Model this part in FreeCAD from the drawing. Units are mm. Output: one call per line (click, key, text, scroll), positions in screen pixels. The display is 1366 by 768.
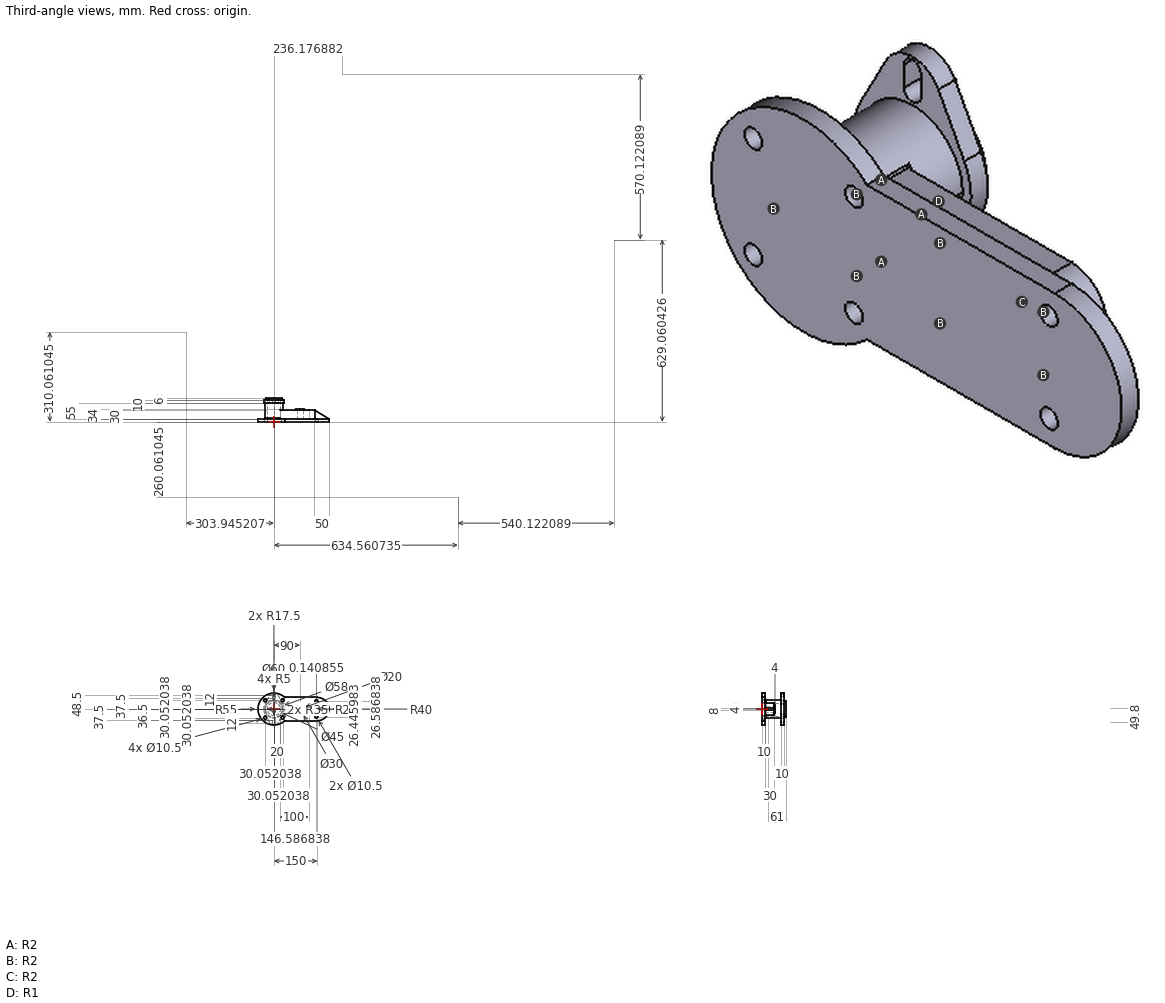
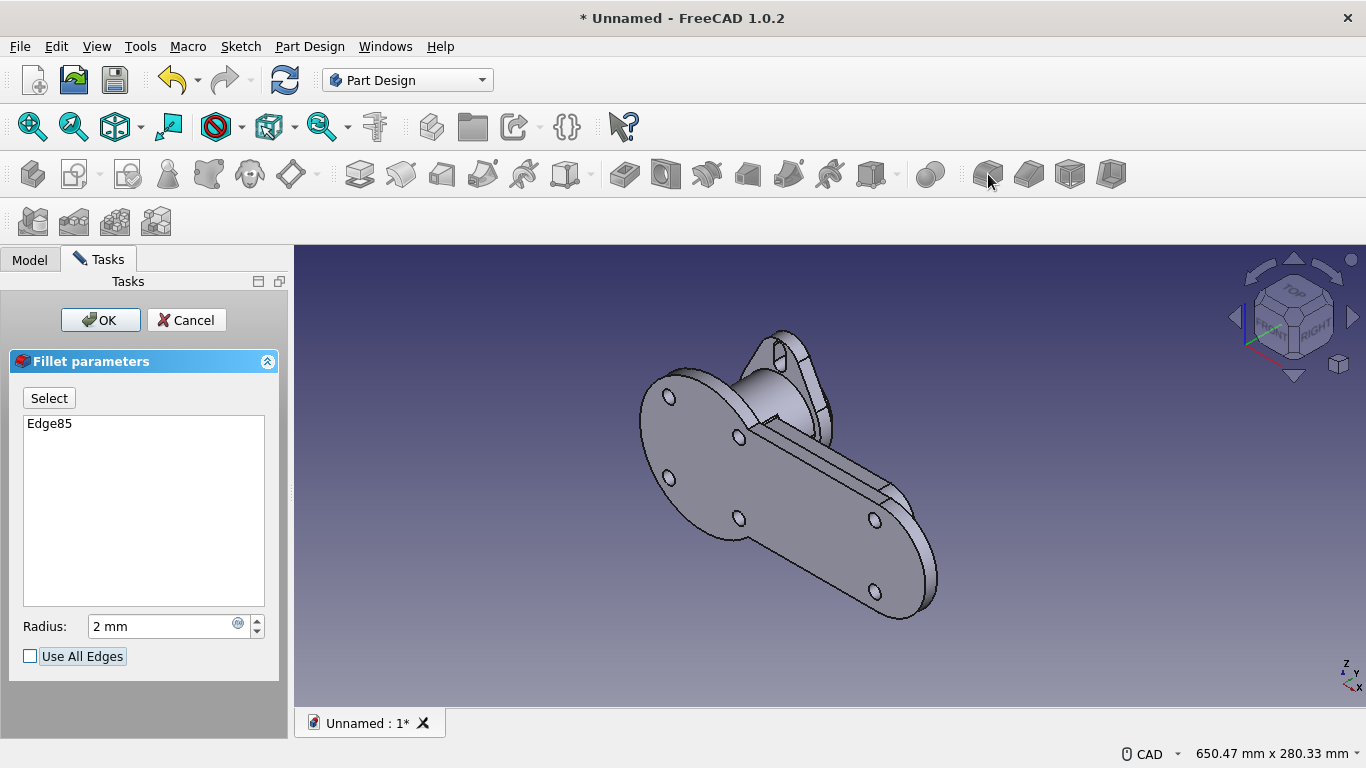
click(101, 320)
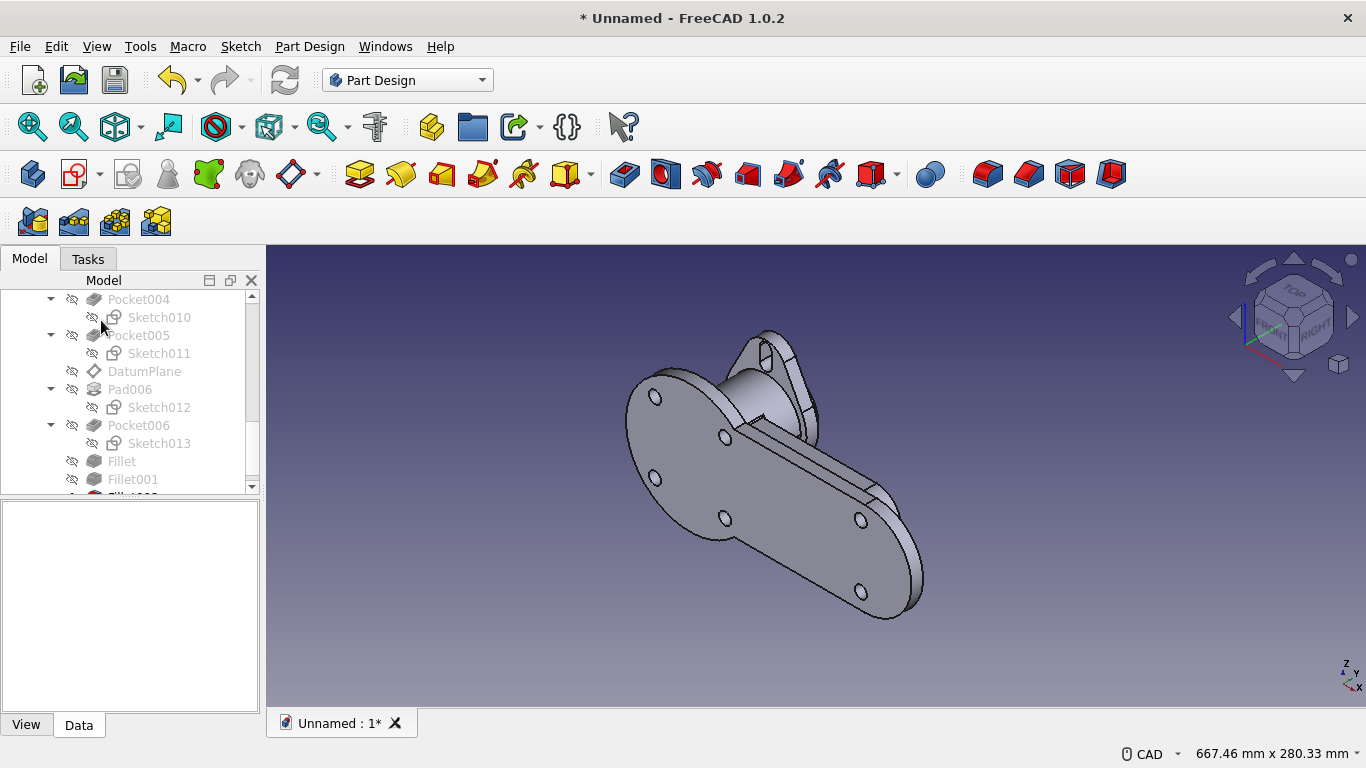
key(2)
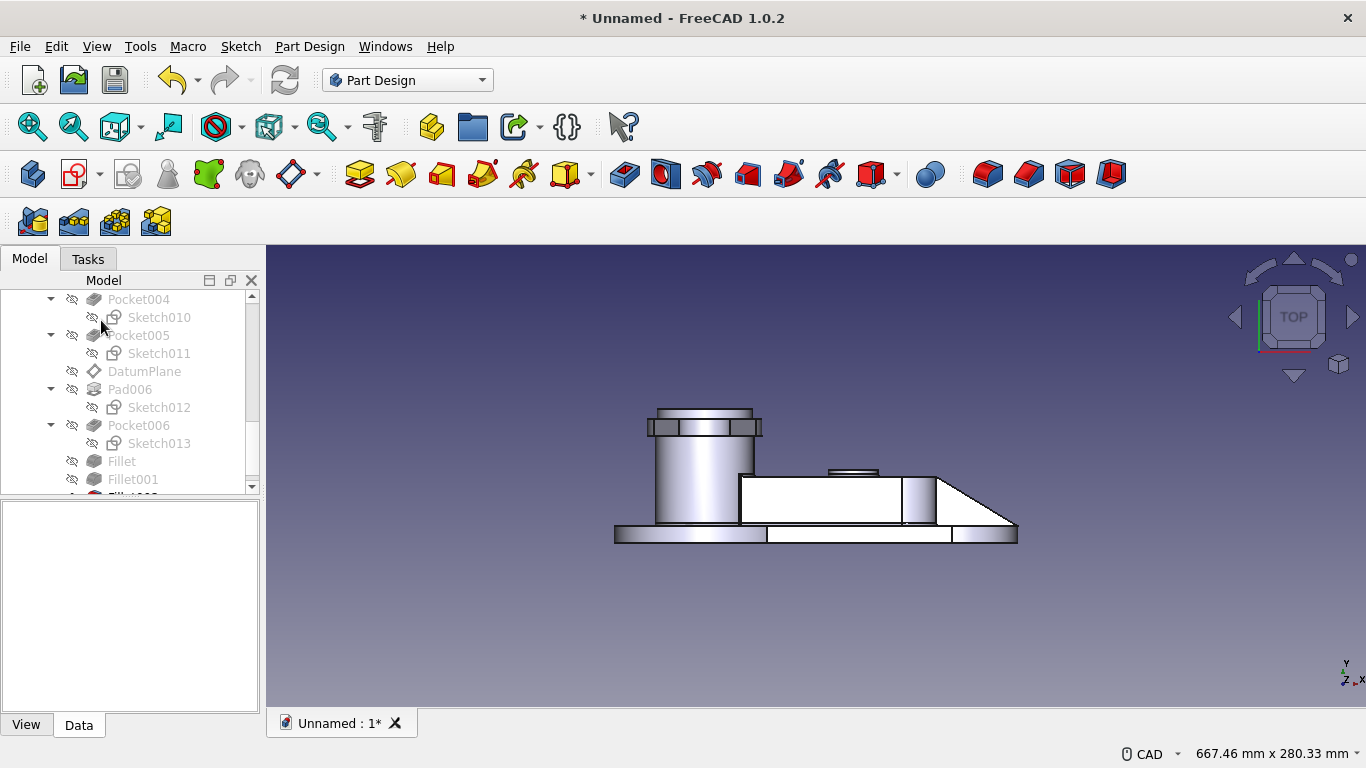
key(v)
key(f)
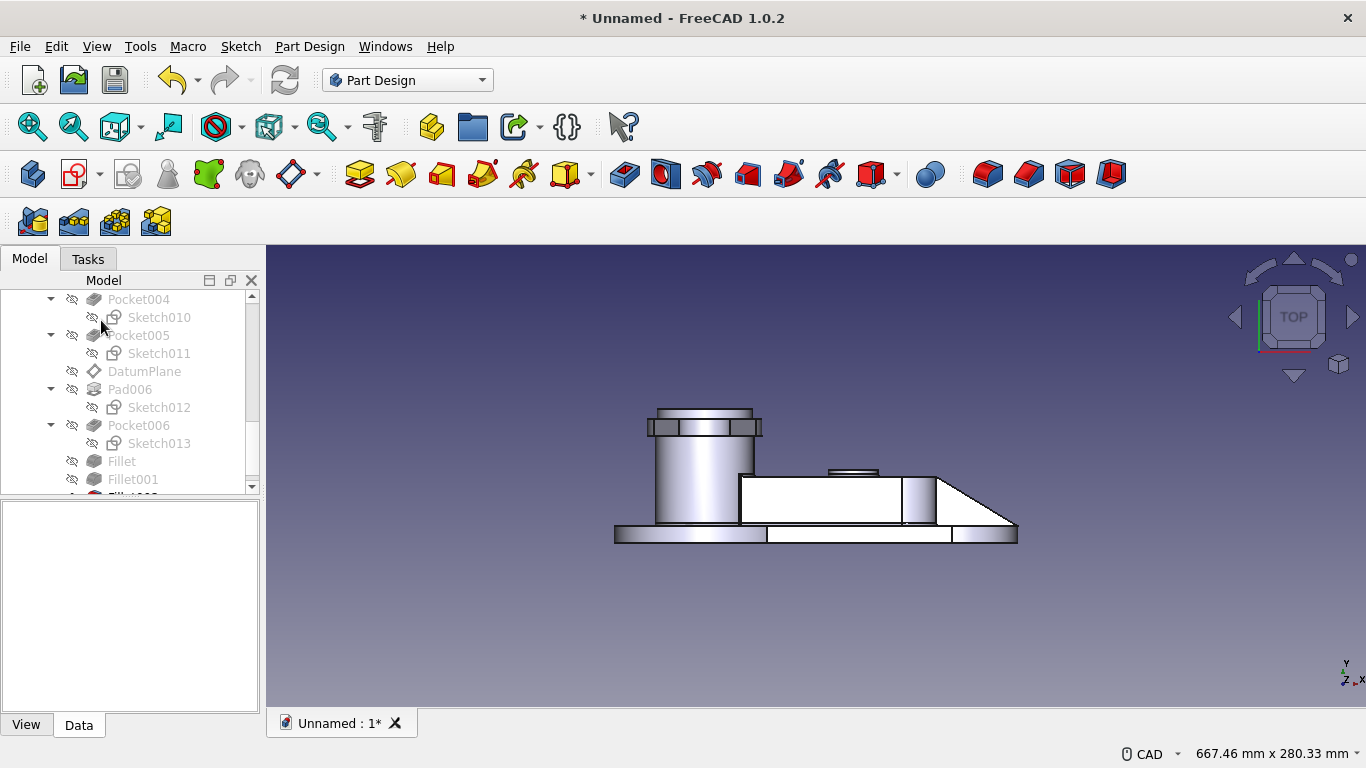
click(666, 408)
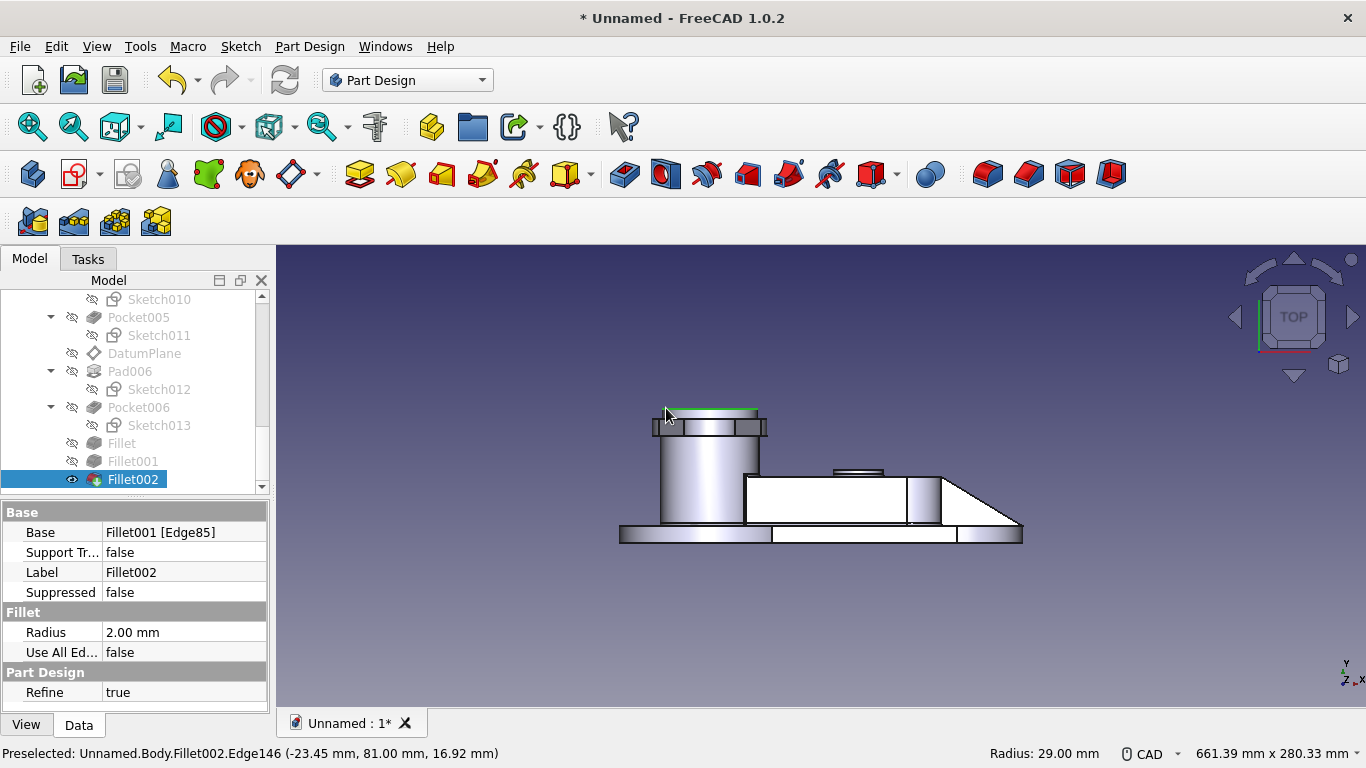
click(988, 174)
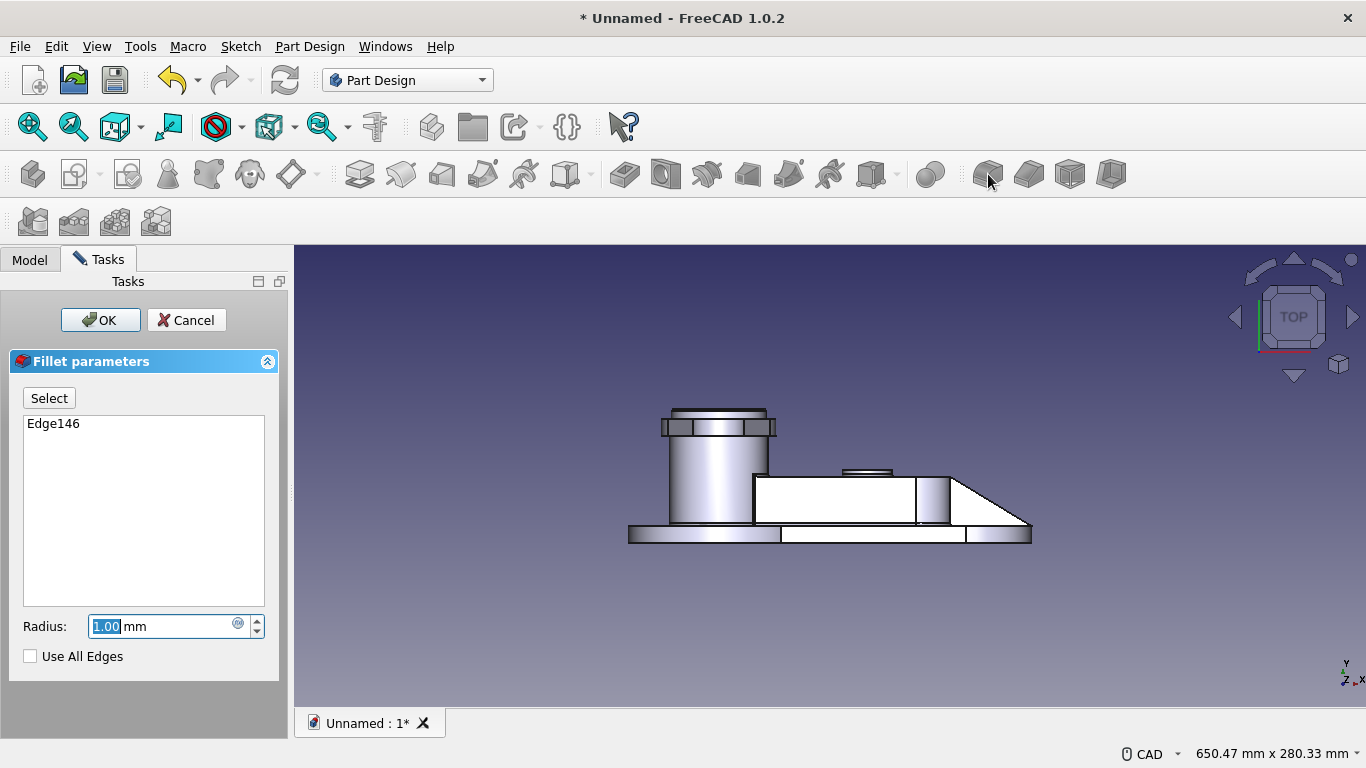
text(1)
key(Tab)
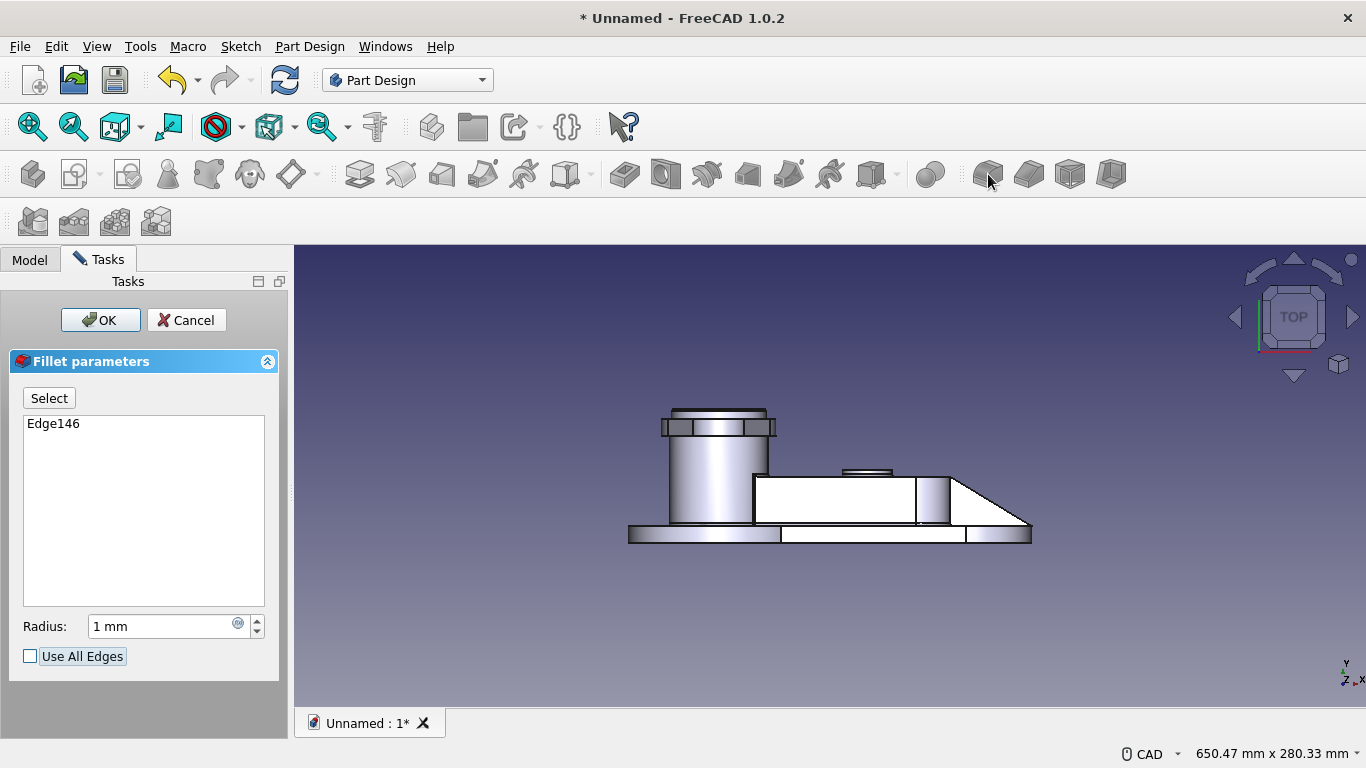
click(101, 320)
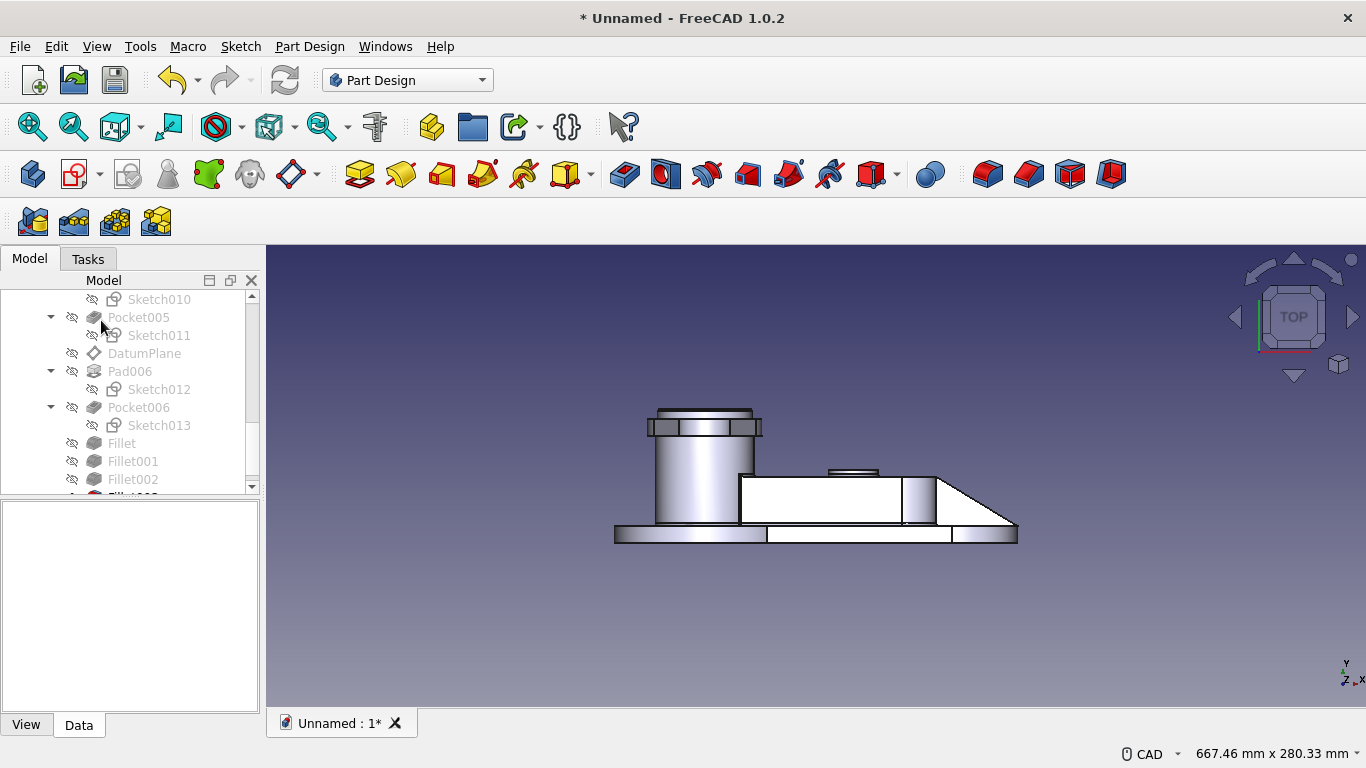
key(0)